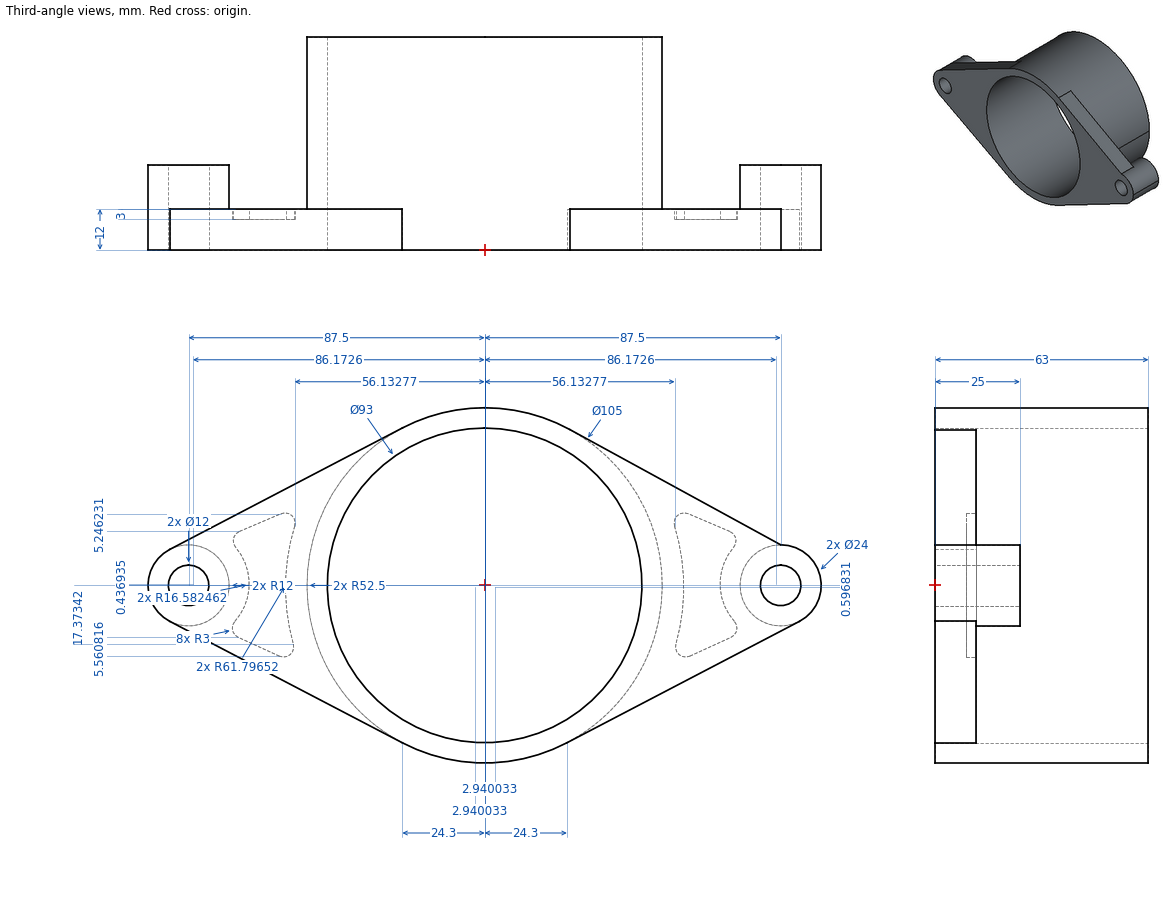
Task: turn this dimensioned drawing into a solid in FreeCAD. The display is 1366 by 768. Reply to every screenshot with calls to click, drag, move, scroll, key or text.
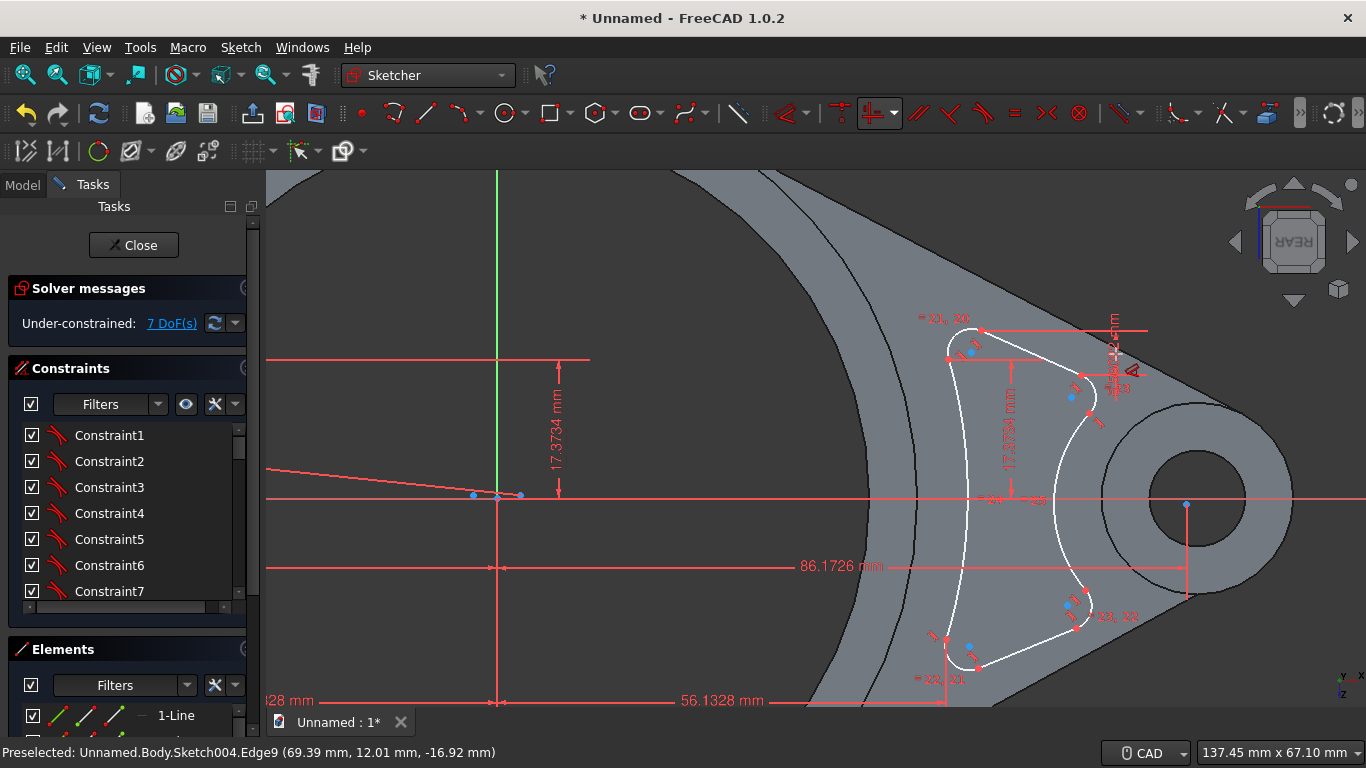
click(1008, 656)
click(1111, 648)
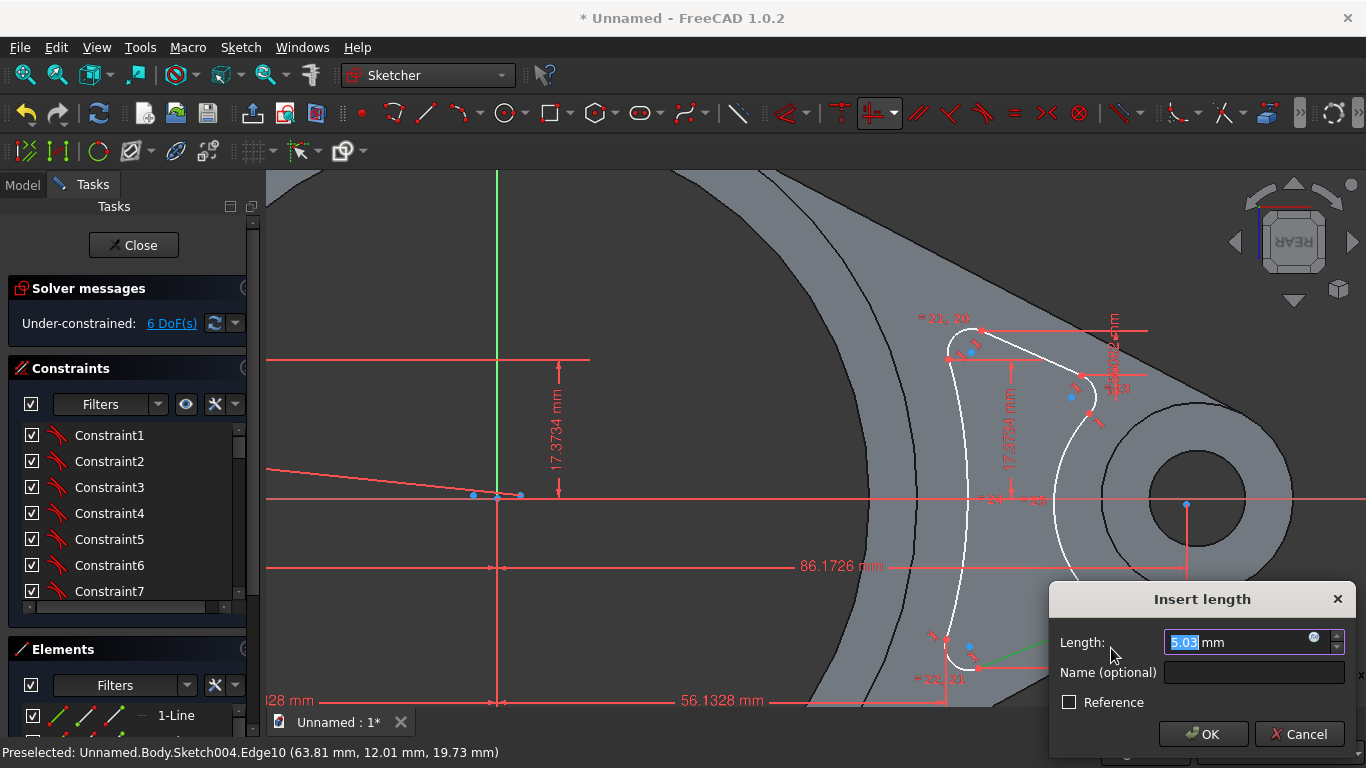
text(5.246231)
key(Return)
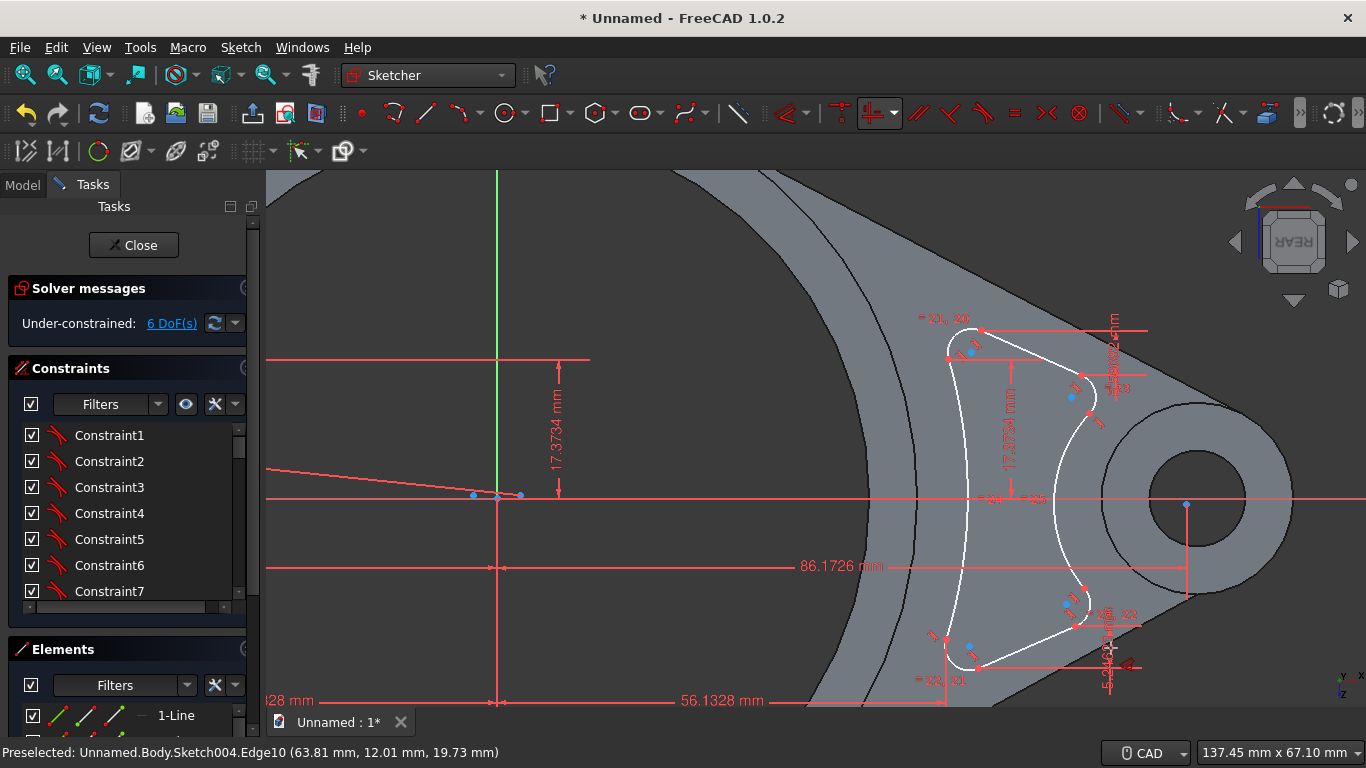
scroll(1052, 364, down, 3)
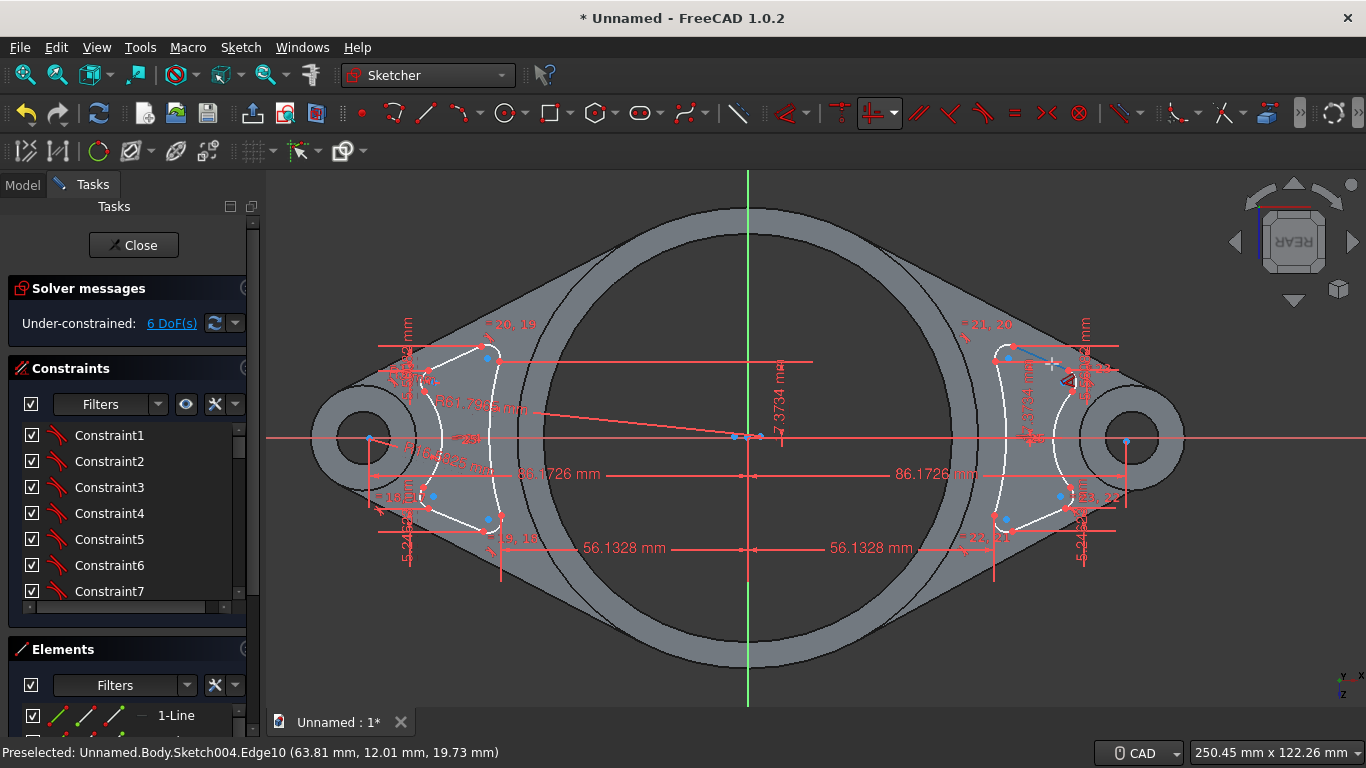
scroll(369, 439, up, 16)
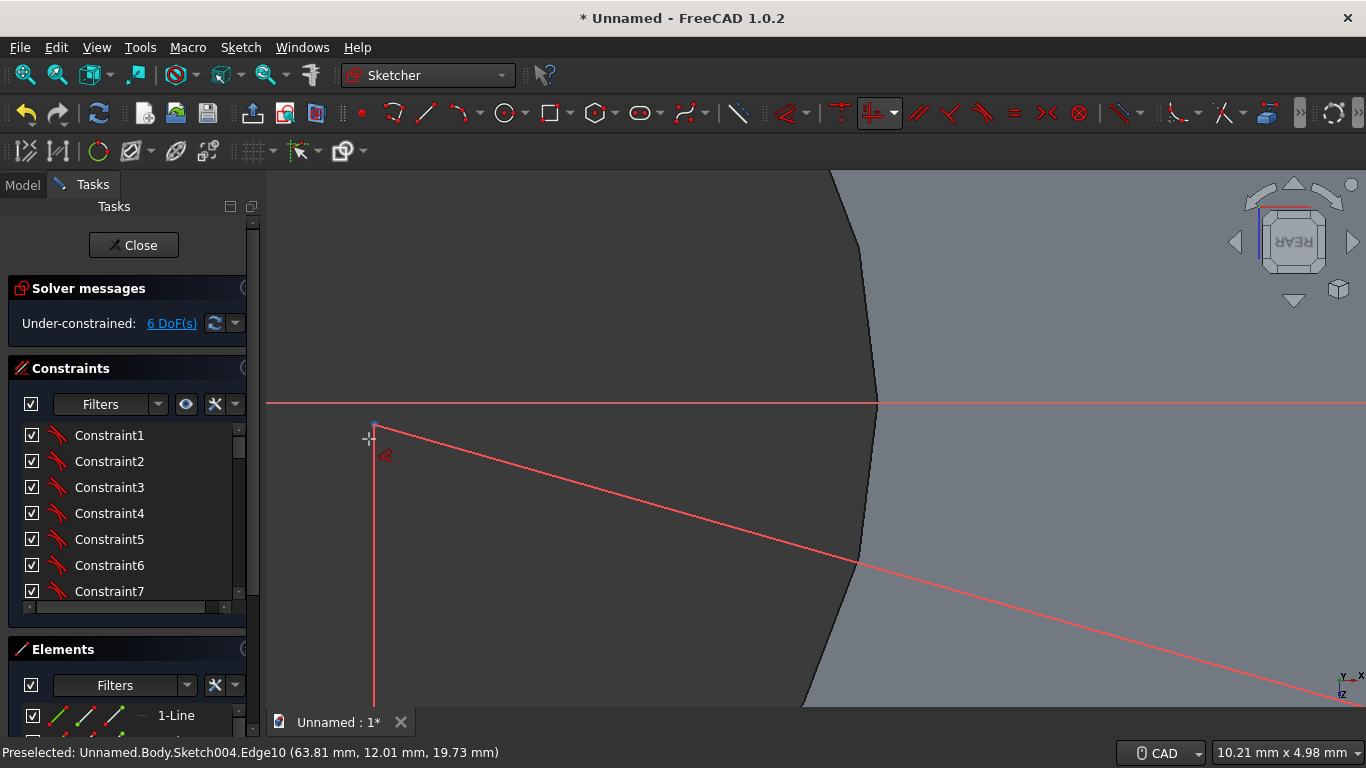
click(374, 425)
click(340, 419)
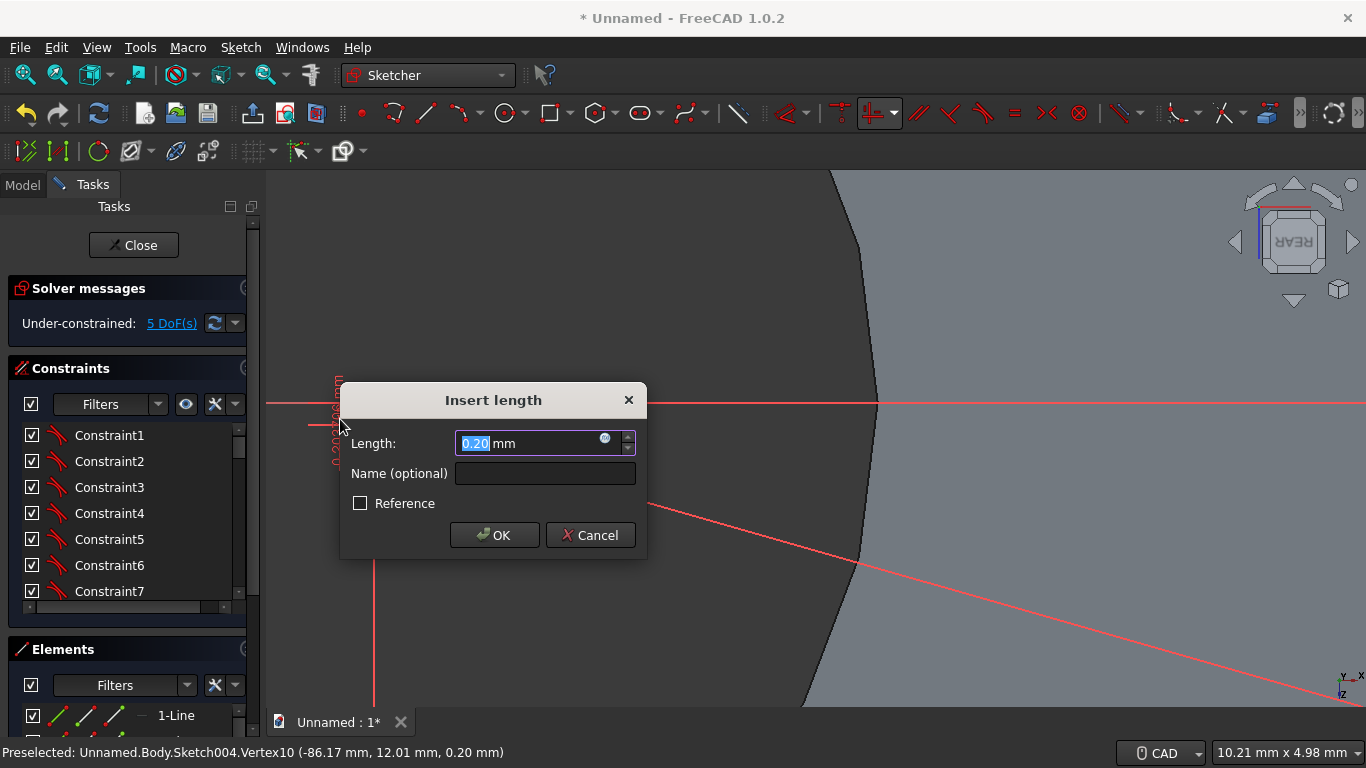
text(0.436935)
key(Return)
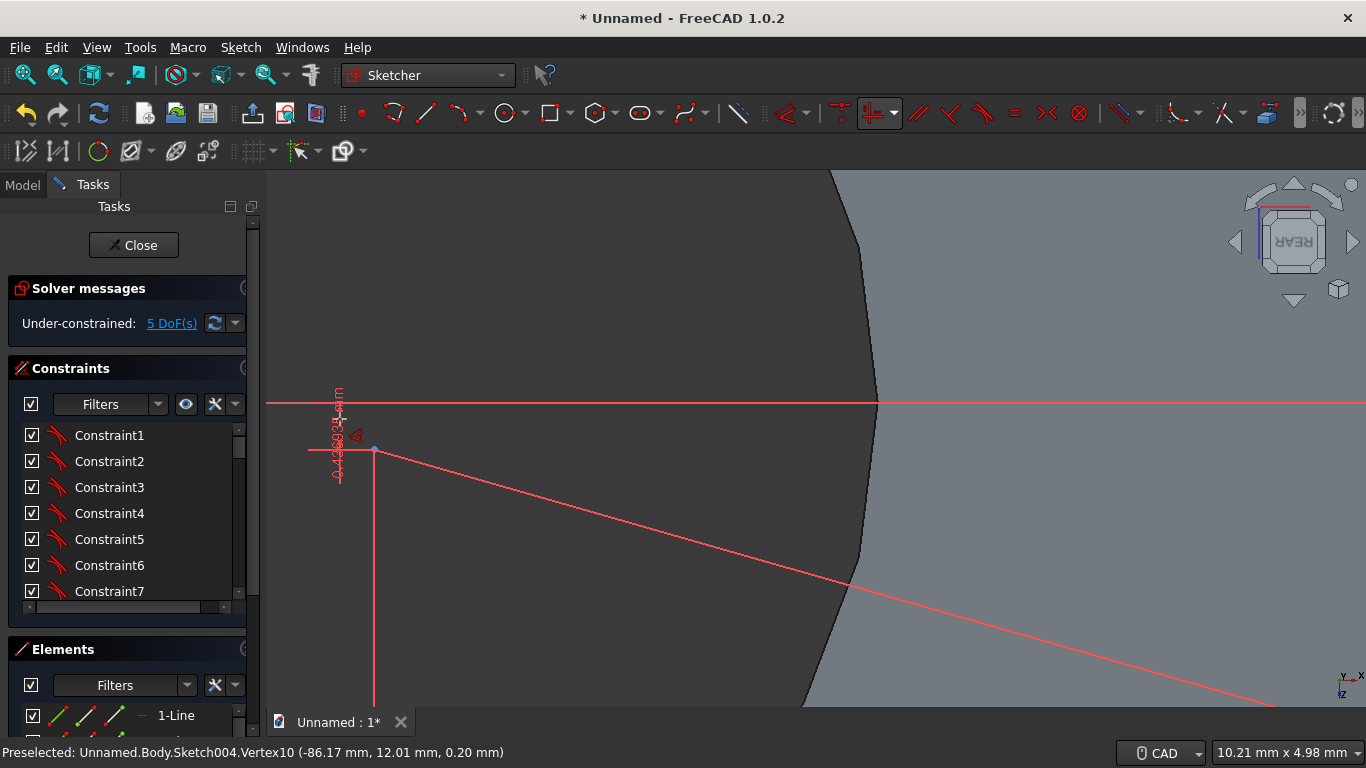
scroll(294, 440, down, 15)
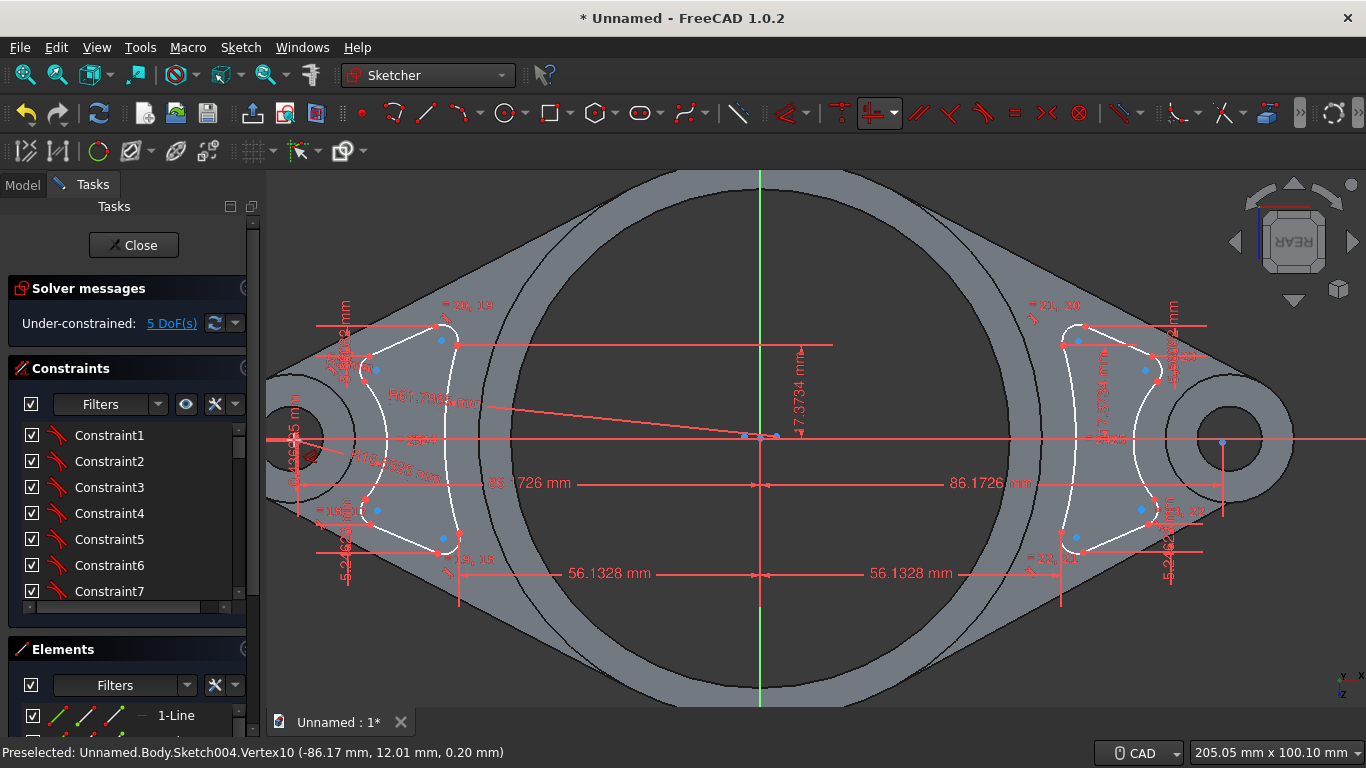
scroll(776, 436, up, 5)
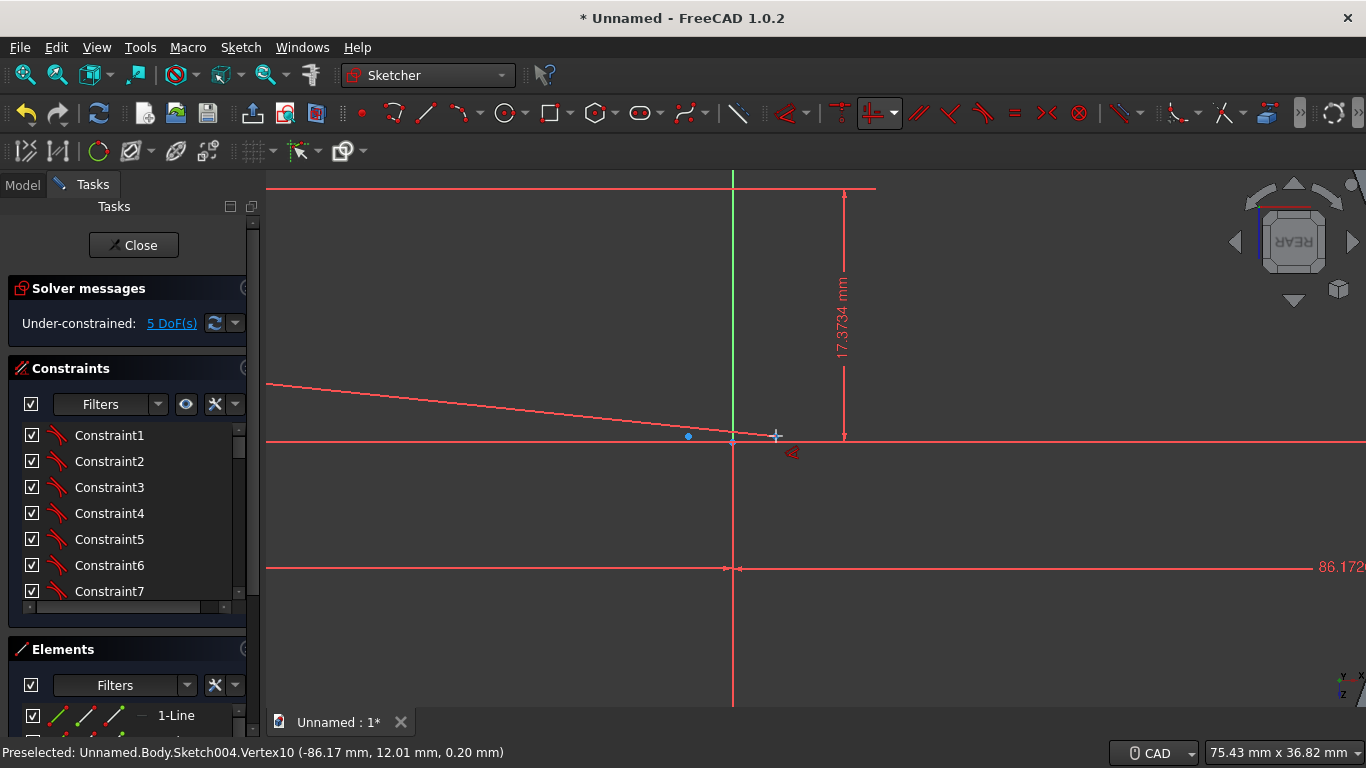
click(776, 436)
click(754, 402)